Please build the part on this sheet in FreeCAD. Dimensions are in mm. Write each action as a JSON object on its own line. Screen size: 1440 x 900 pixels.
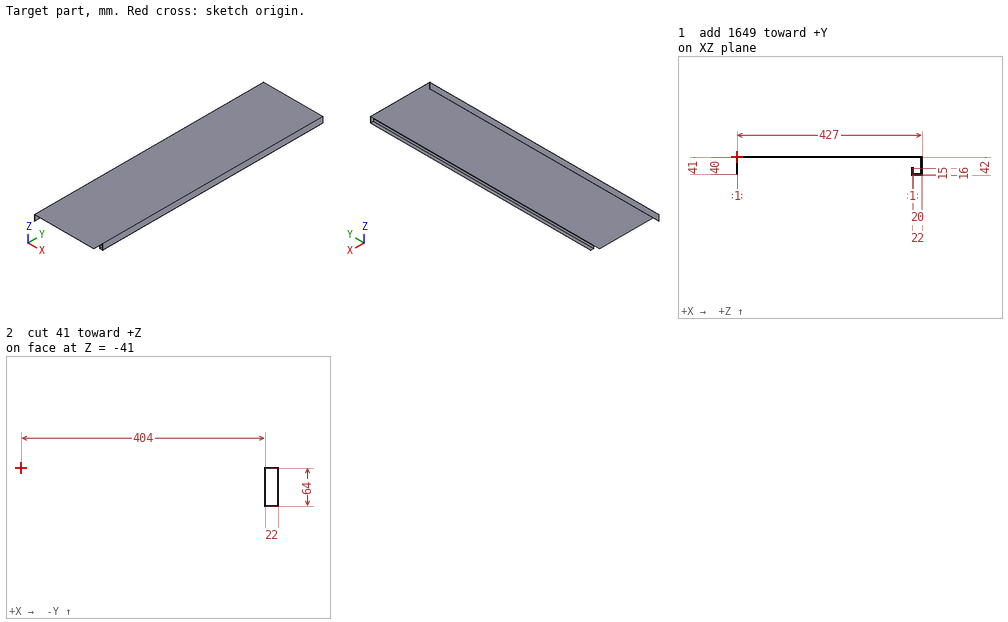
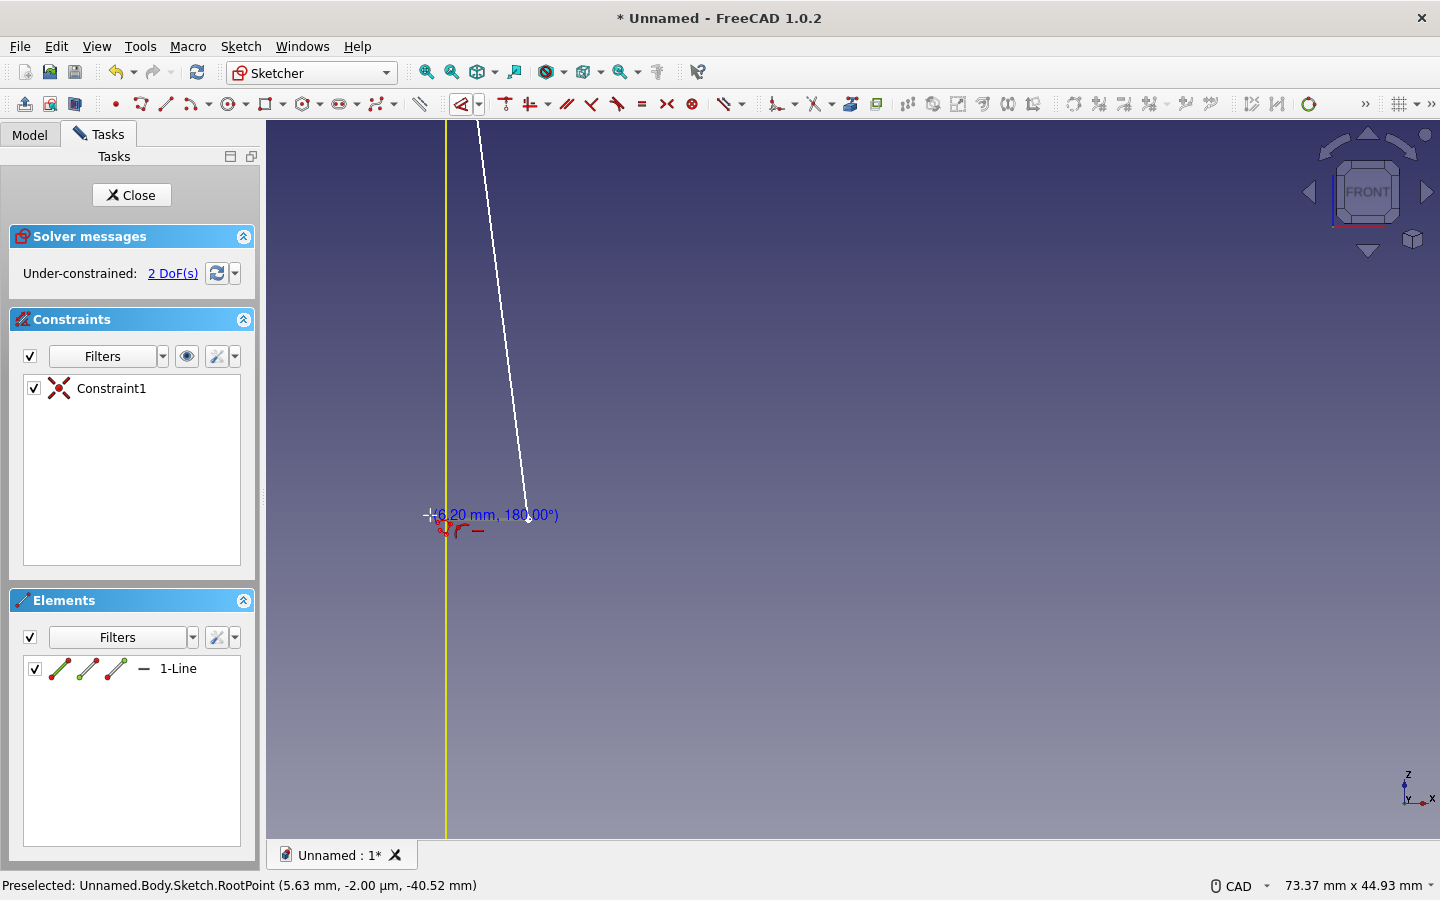
{"action": "left_click", "coordinate": [430, 511]}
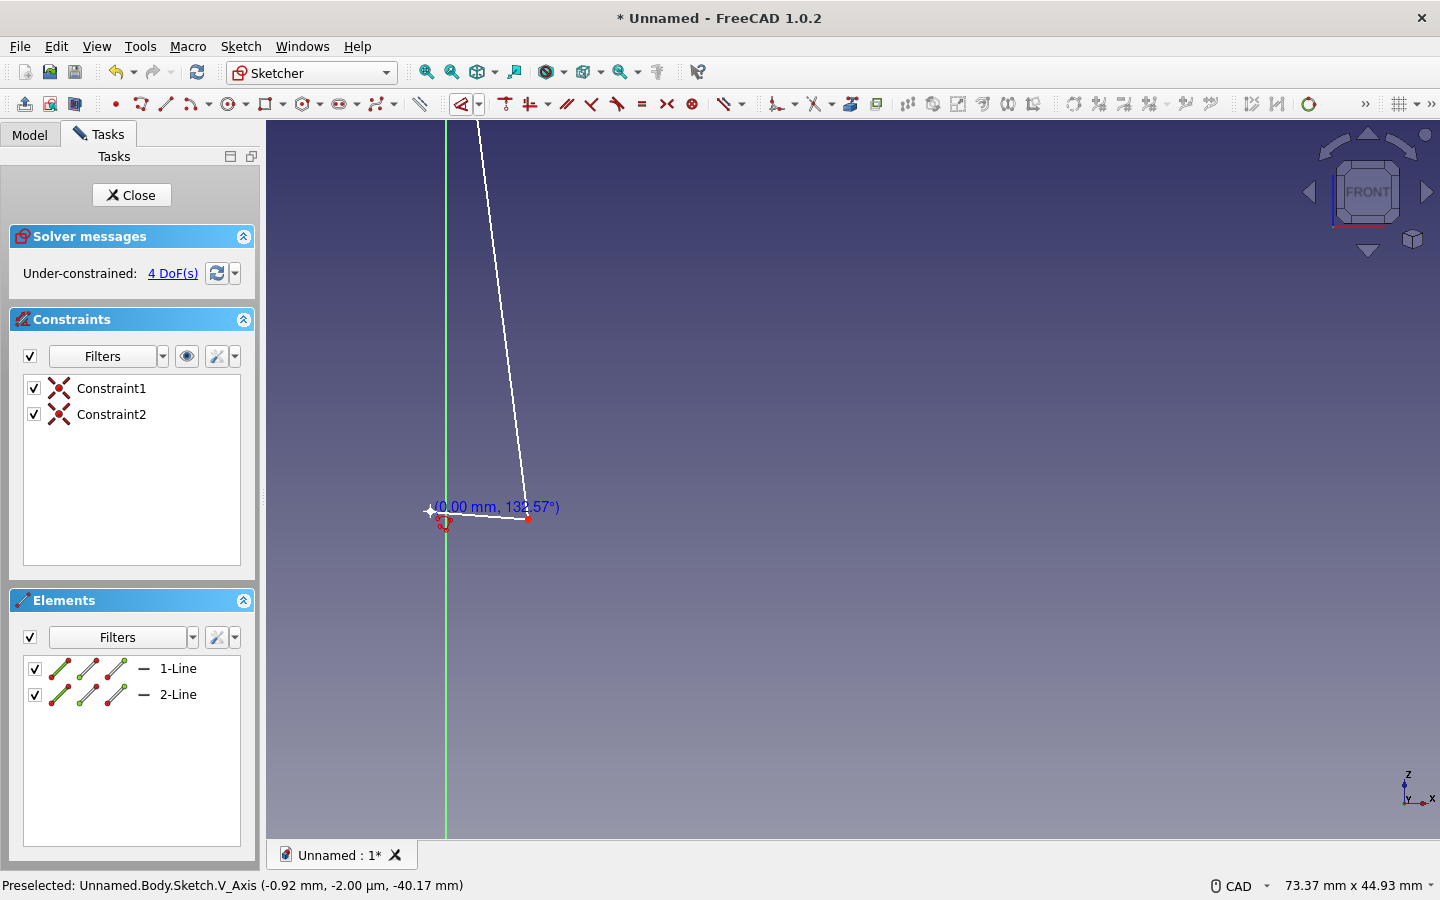
{"action": "scroll", "coordinate": [403, 516], "scroll_direction": "down", "scroll_amount": 11}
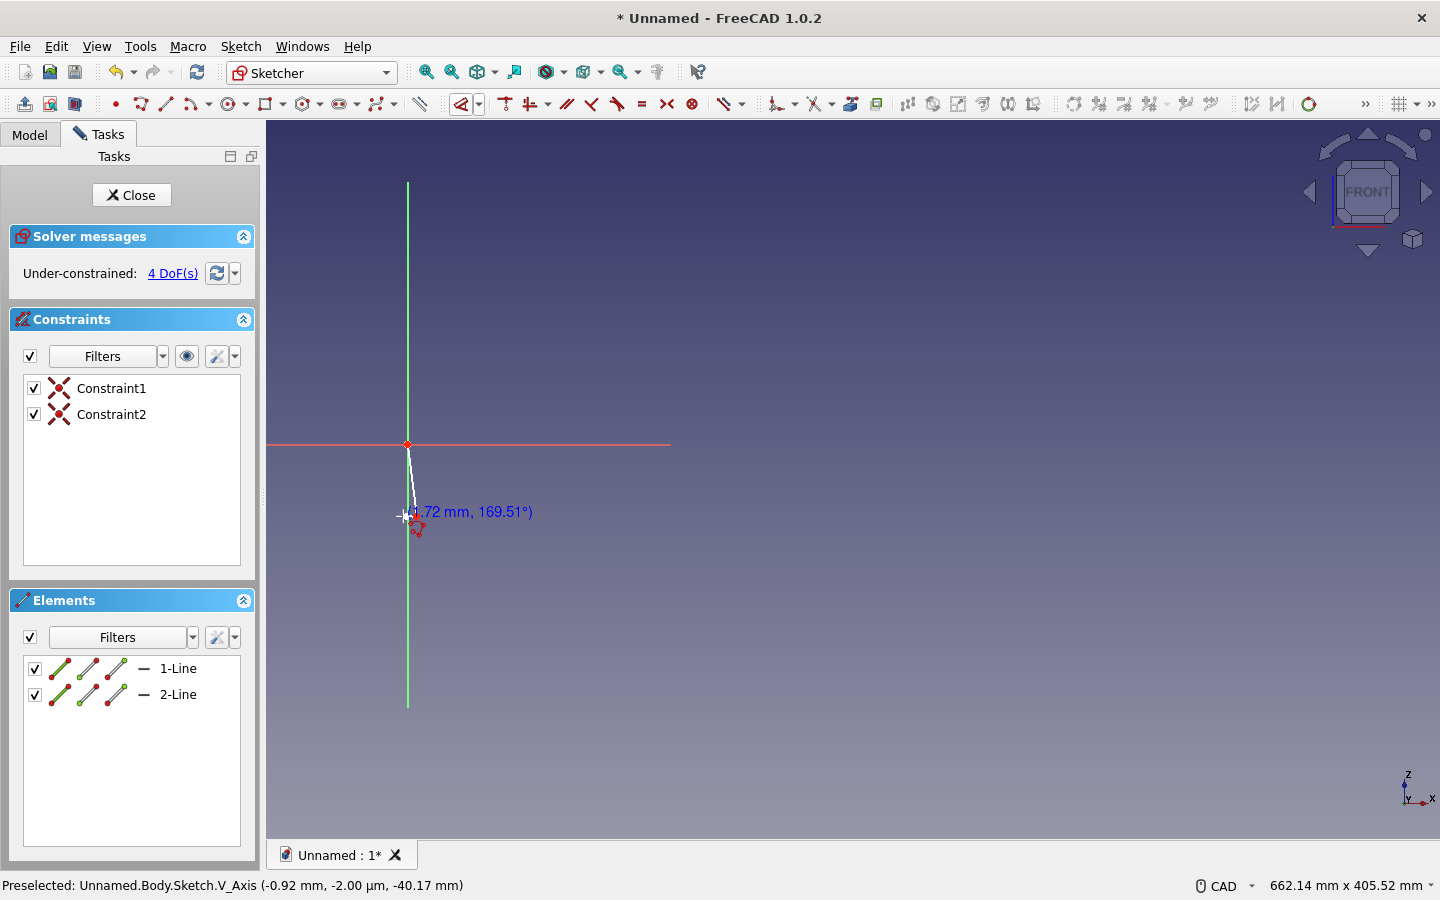
{"action": "scroll", "coordinate": [406, 443], "scroll_direction": "up", "scroll_amount": 11}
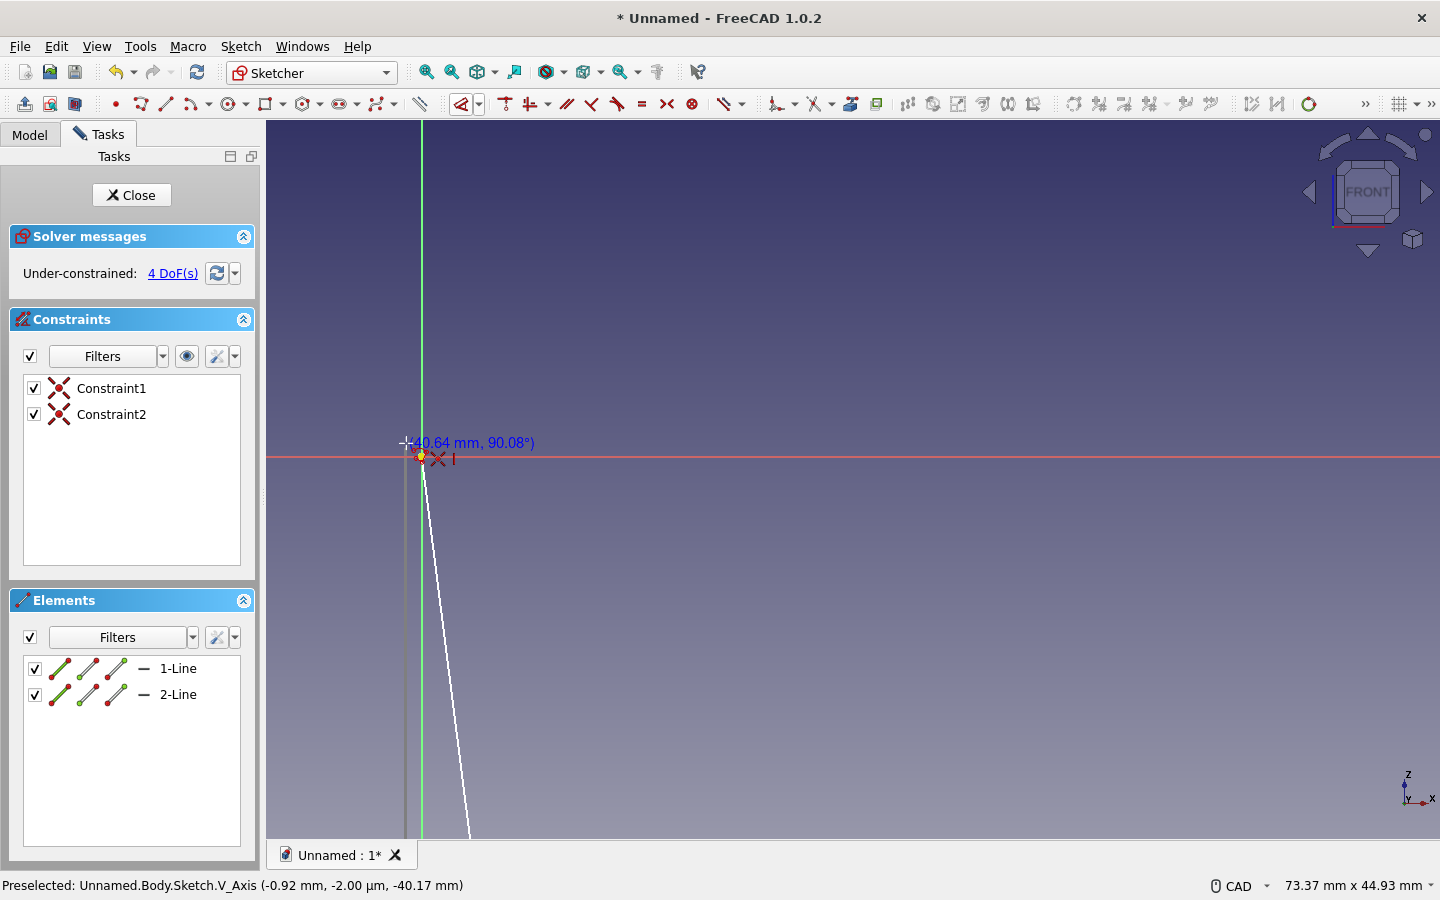
{"action": "left_click", "coordinate": [406, 441]}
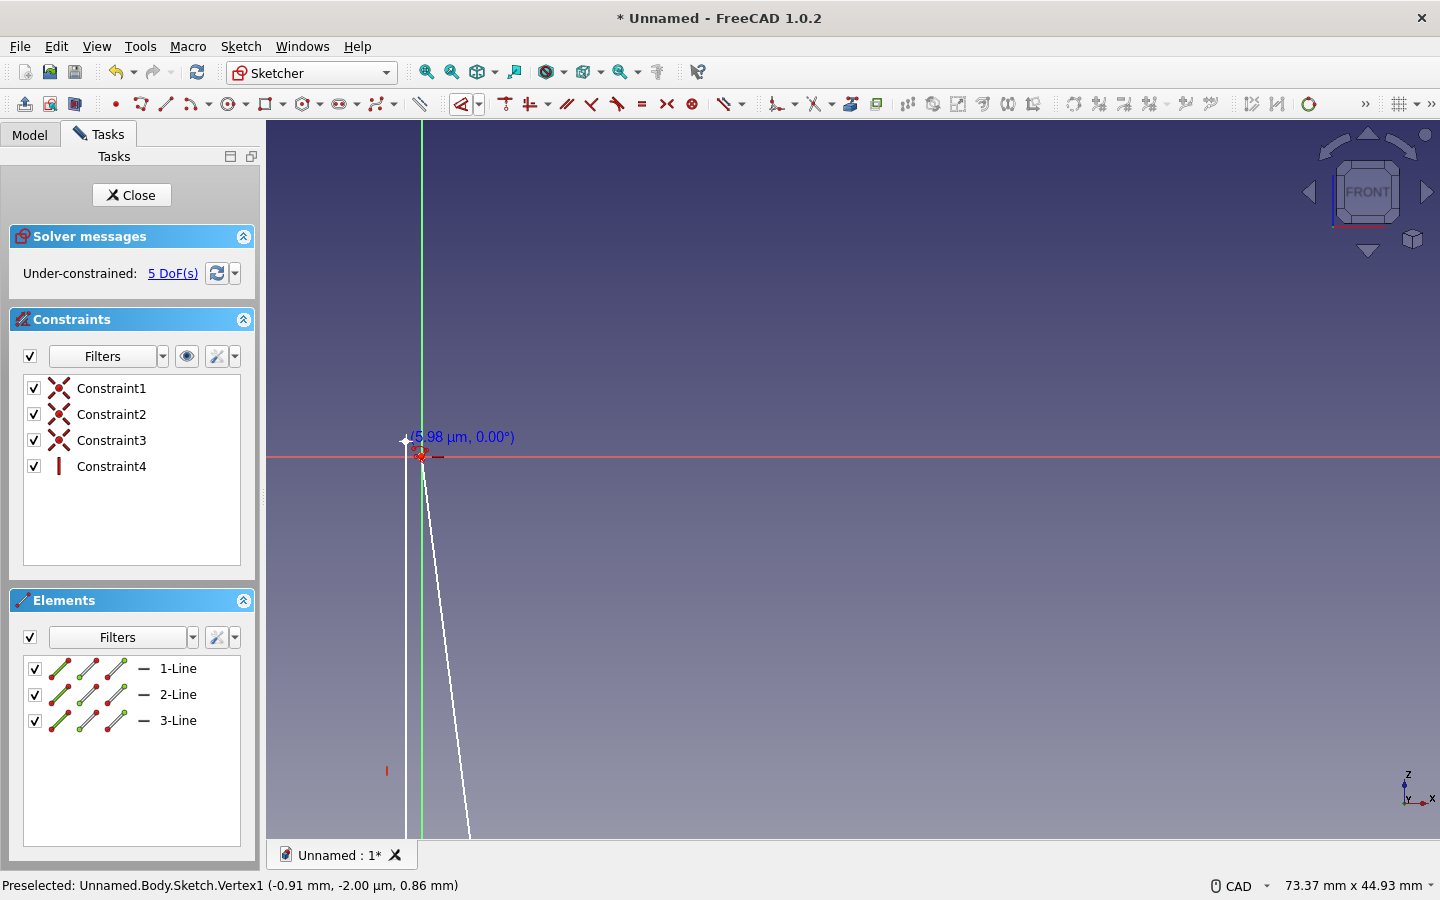
{"action": "scroll", "coordinate": [406, 442], "scroll_direction": "down", "scroll_amount": 11}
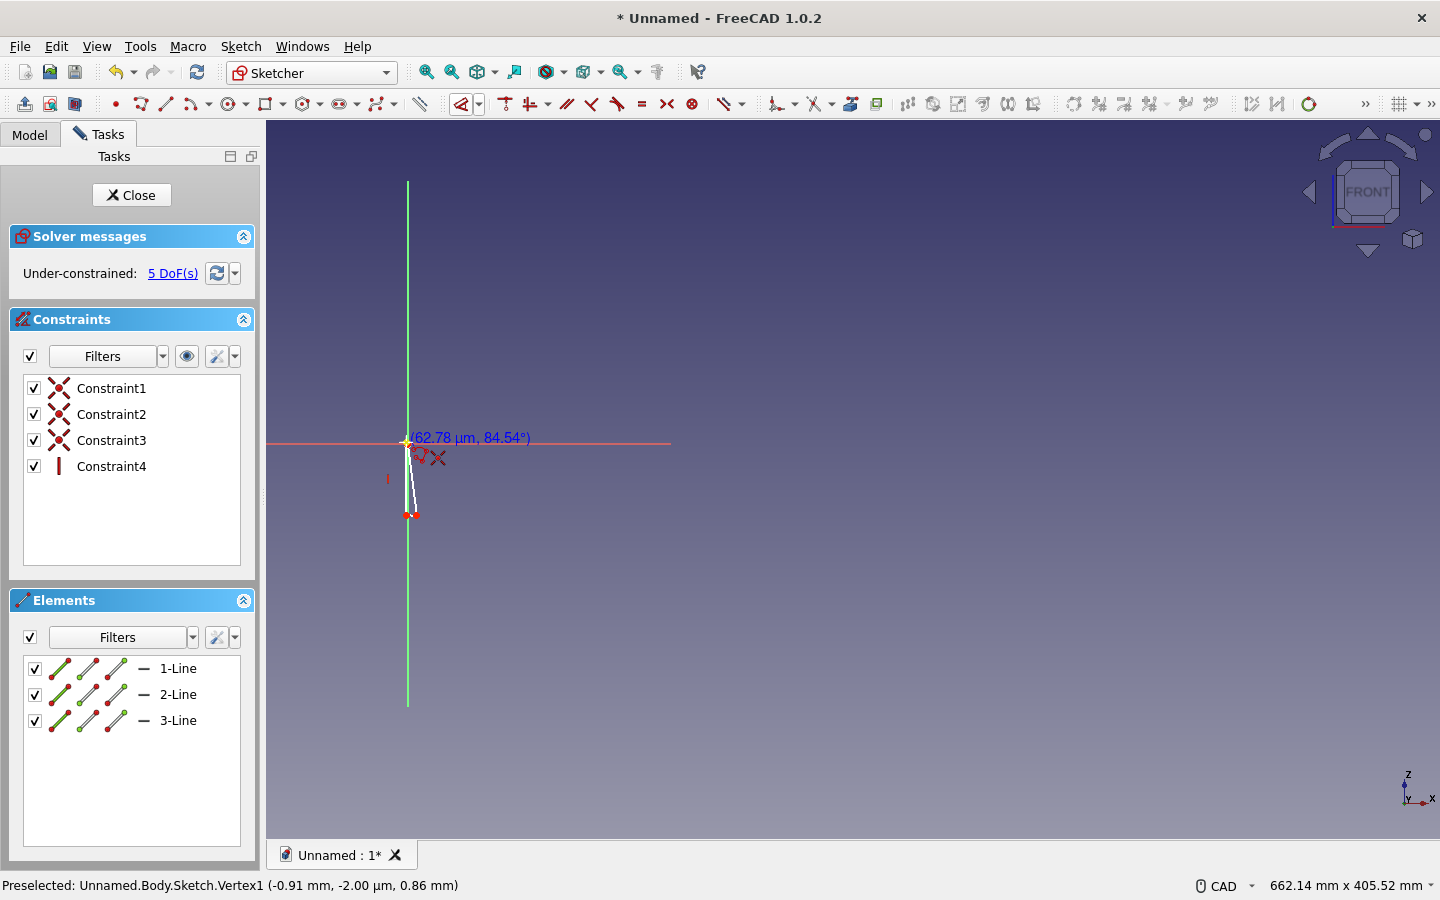
{"action": "scroll", "coordinate": [1163, 442], "scroll_direction": "up", "scroll_amount": 11}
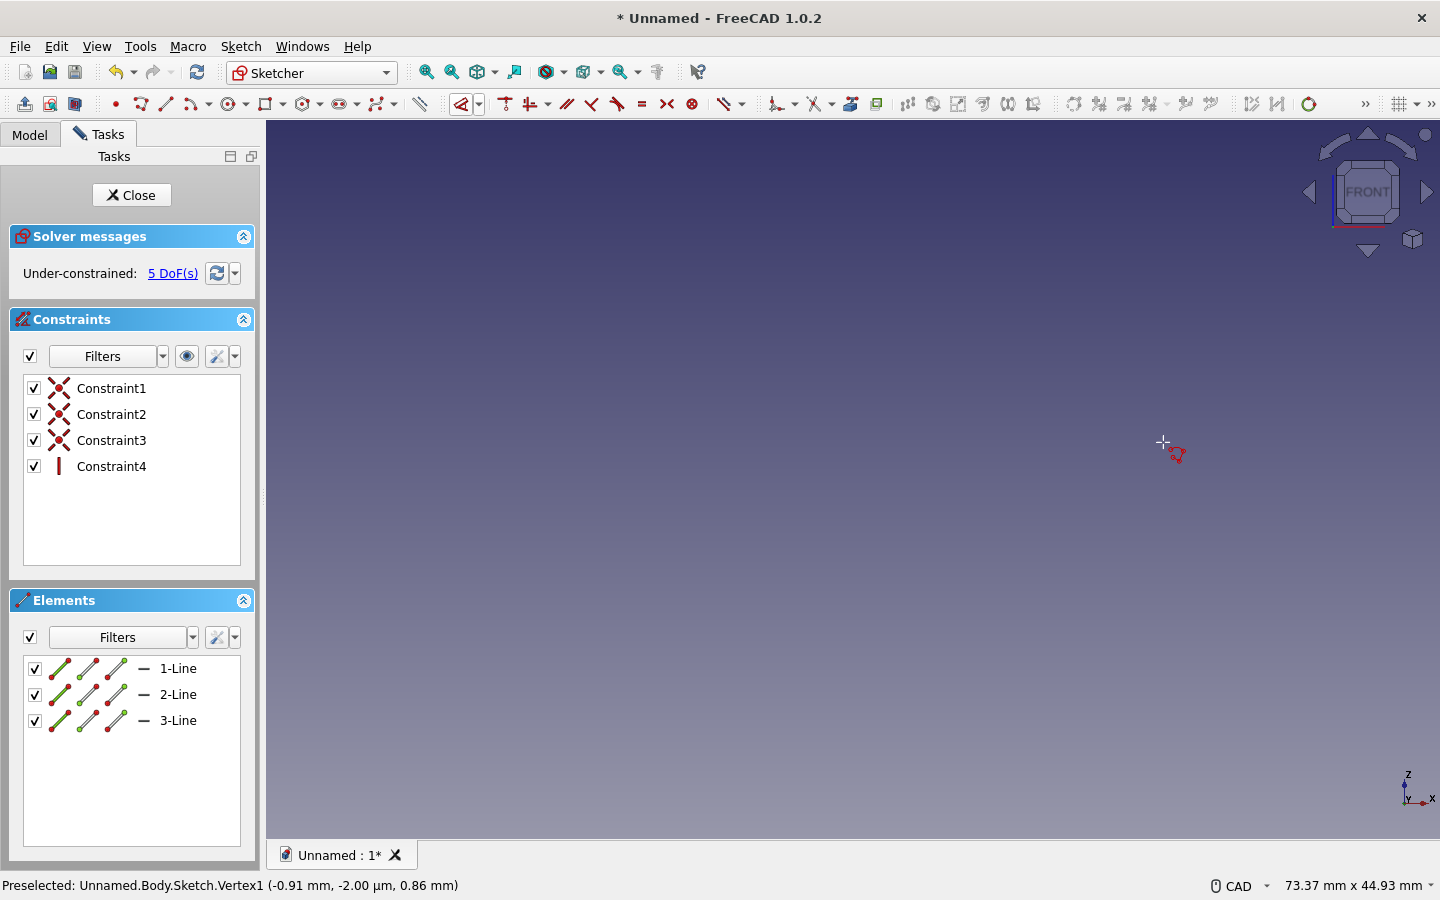
{"action": "left_click", "coordinate": [1158, 441]}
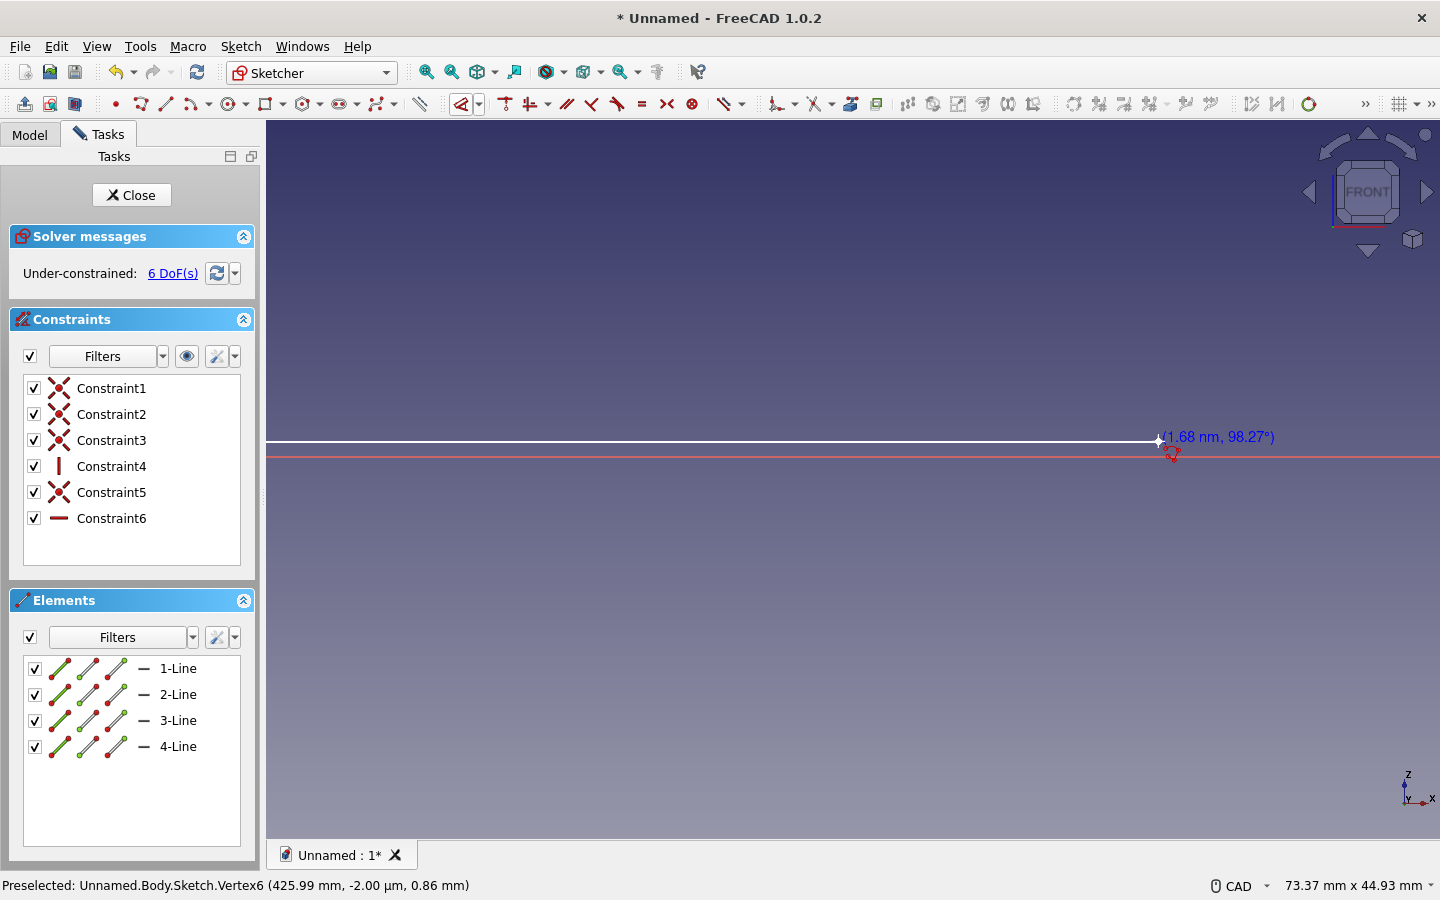
{"action": "scroll", "coordinate": [1164, 442], "scroll_direction": "down", "scroll_amount": 11}